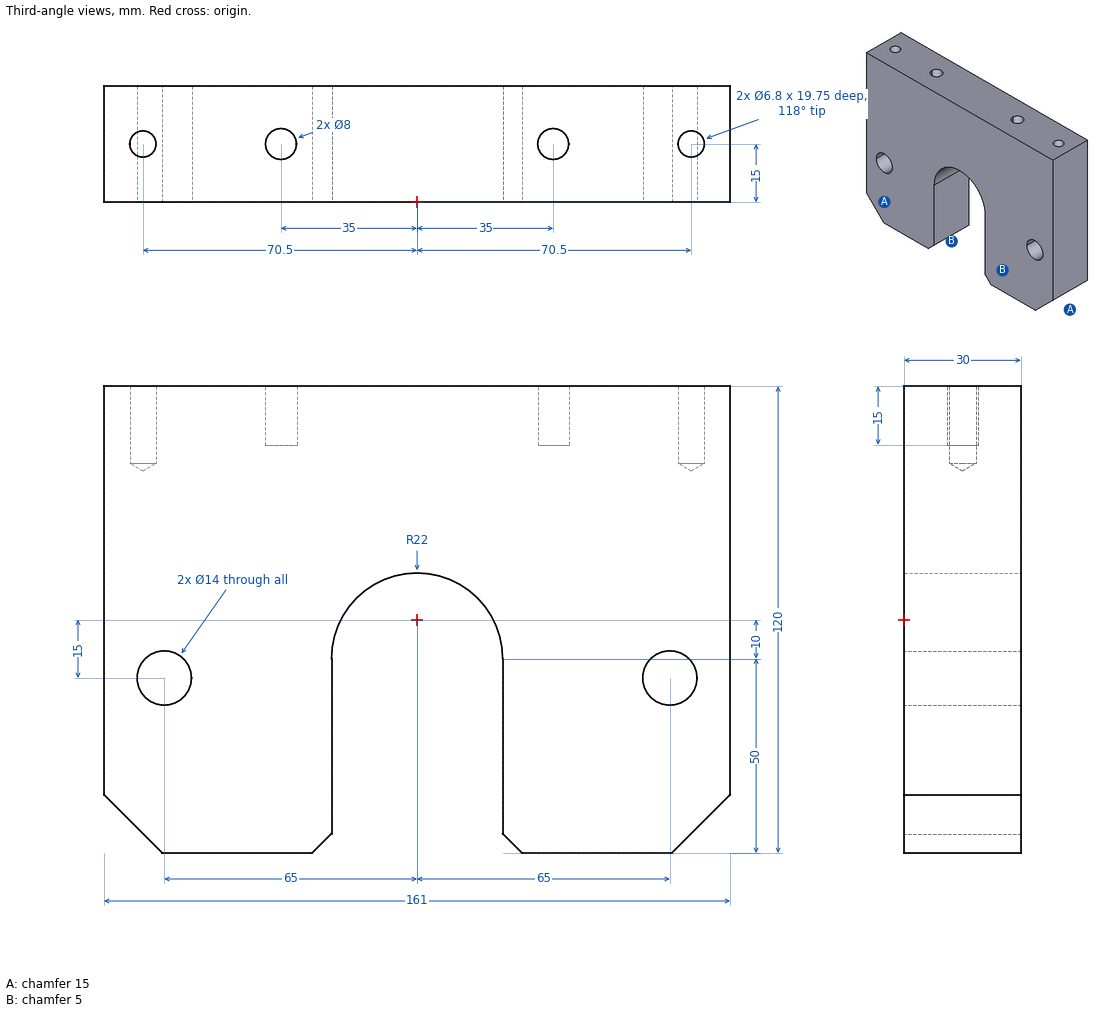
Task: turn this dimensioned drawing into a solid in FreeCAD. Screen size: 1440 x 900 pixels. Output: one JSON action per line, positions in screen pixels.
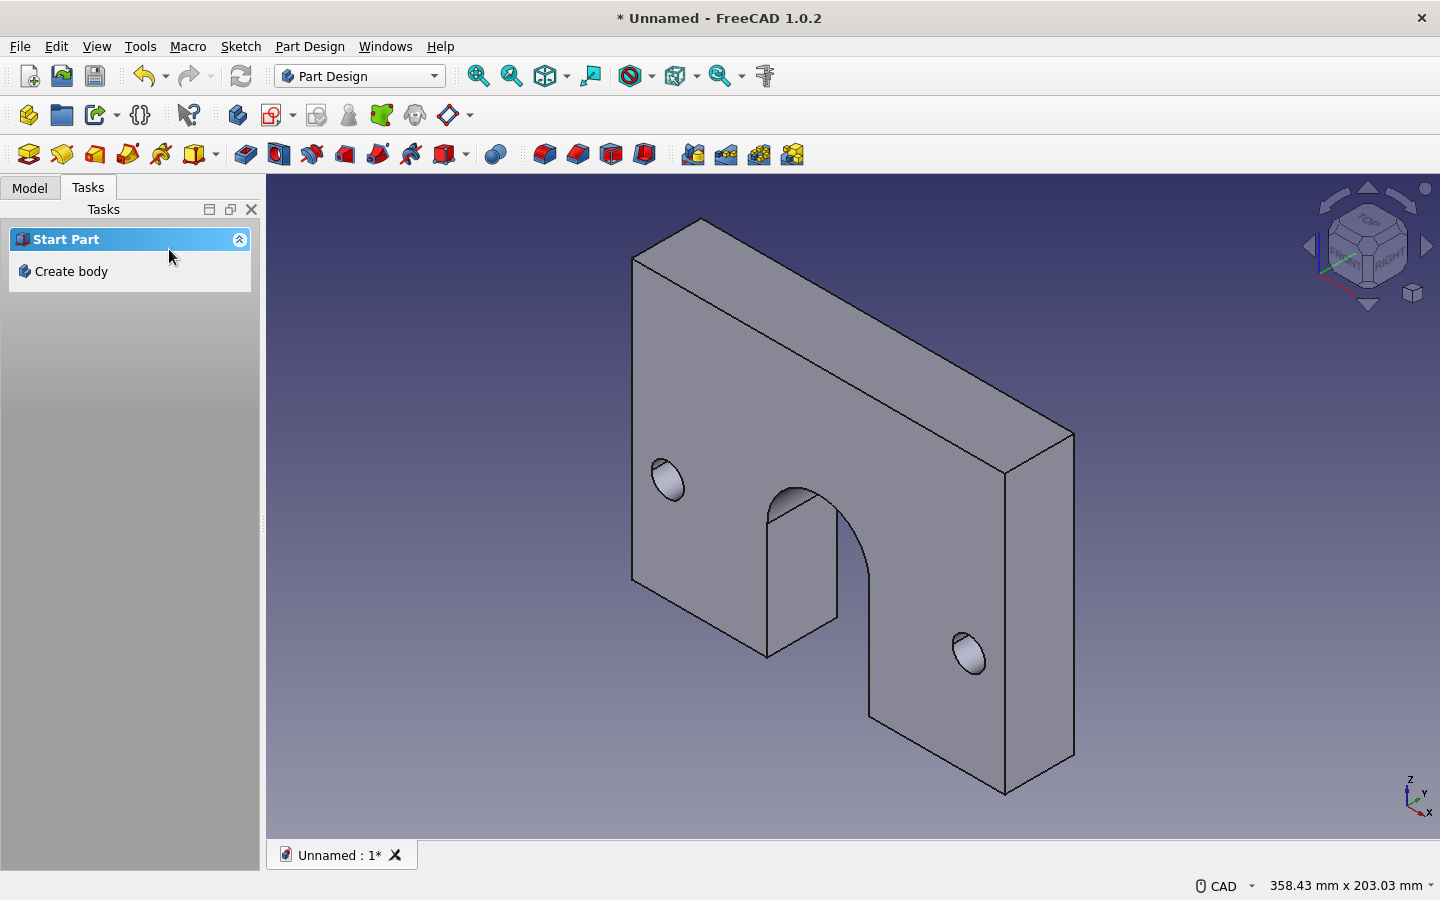
{"action": "left_click", "coordinate": [960, 407]}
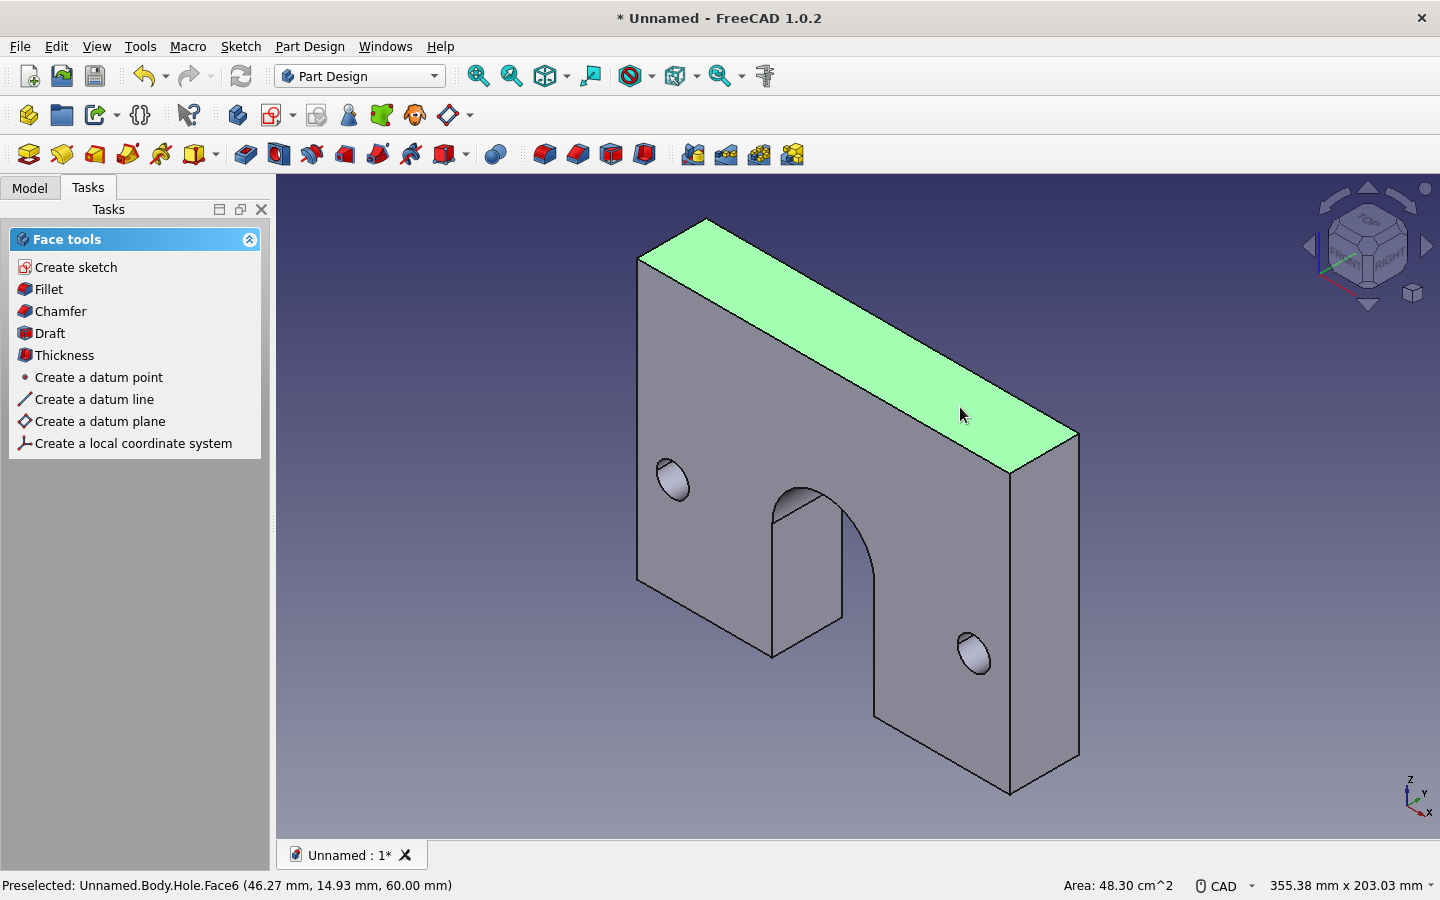
{"action": "left_click", "coordinate": [270, 116]}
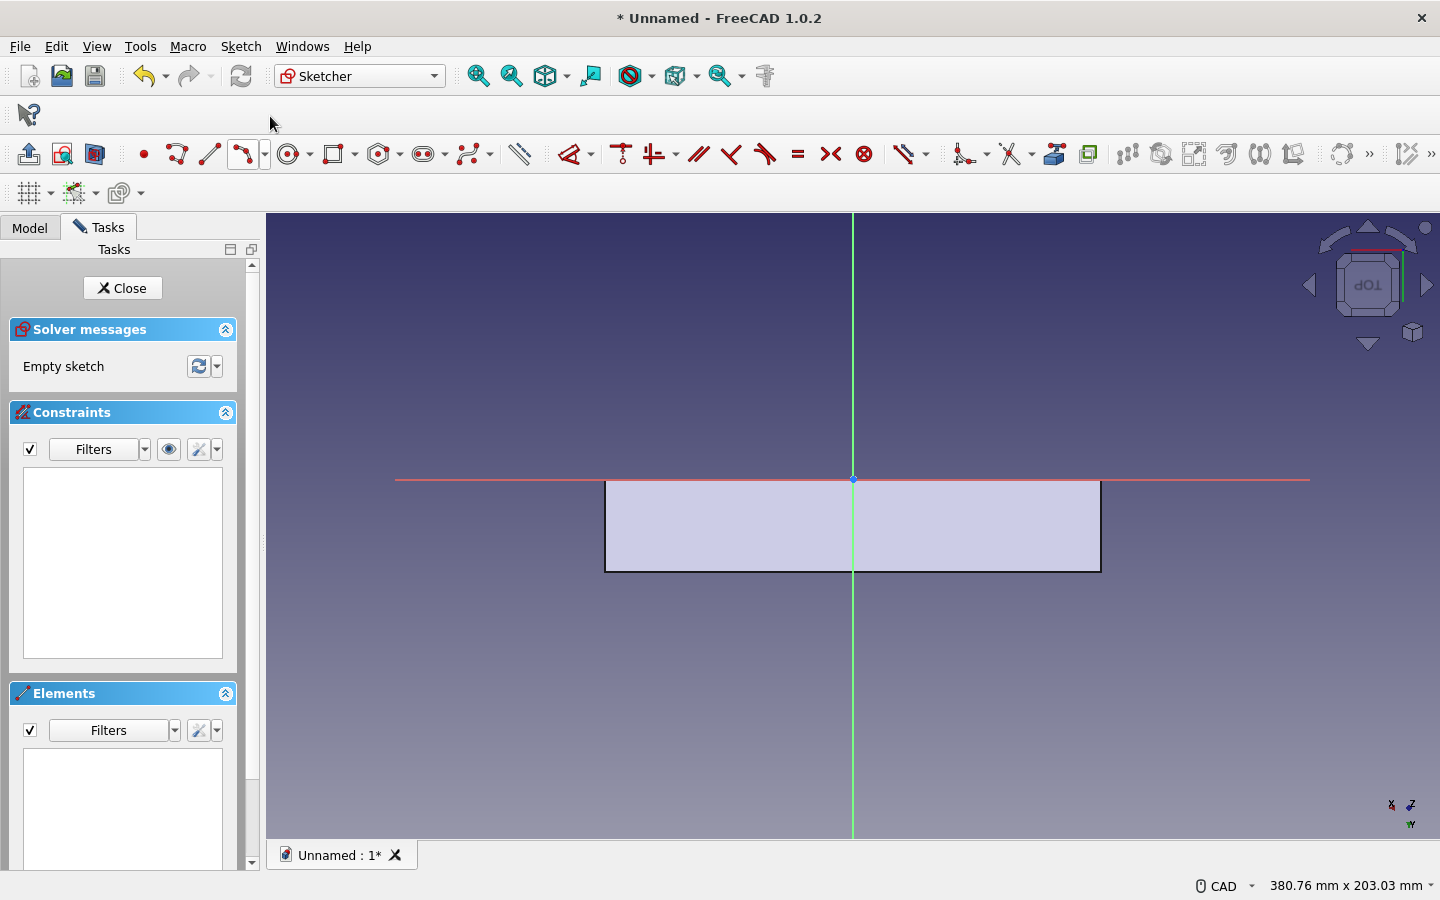
{"action": "scroll", "coordinate": [992, 472], "scroll_direction": "up", "scroll_amount": 2}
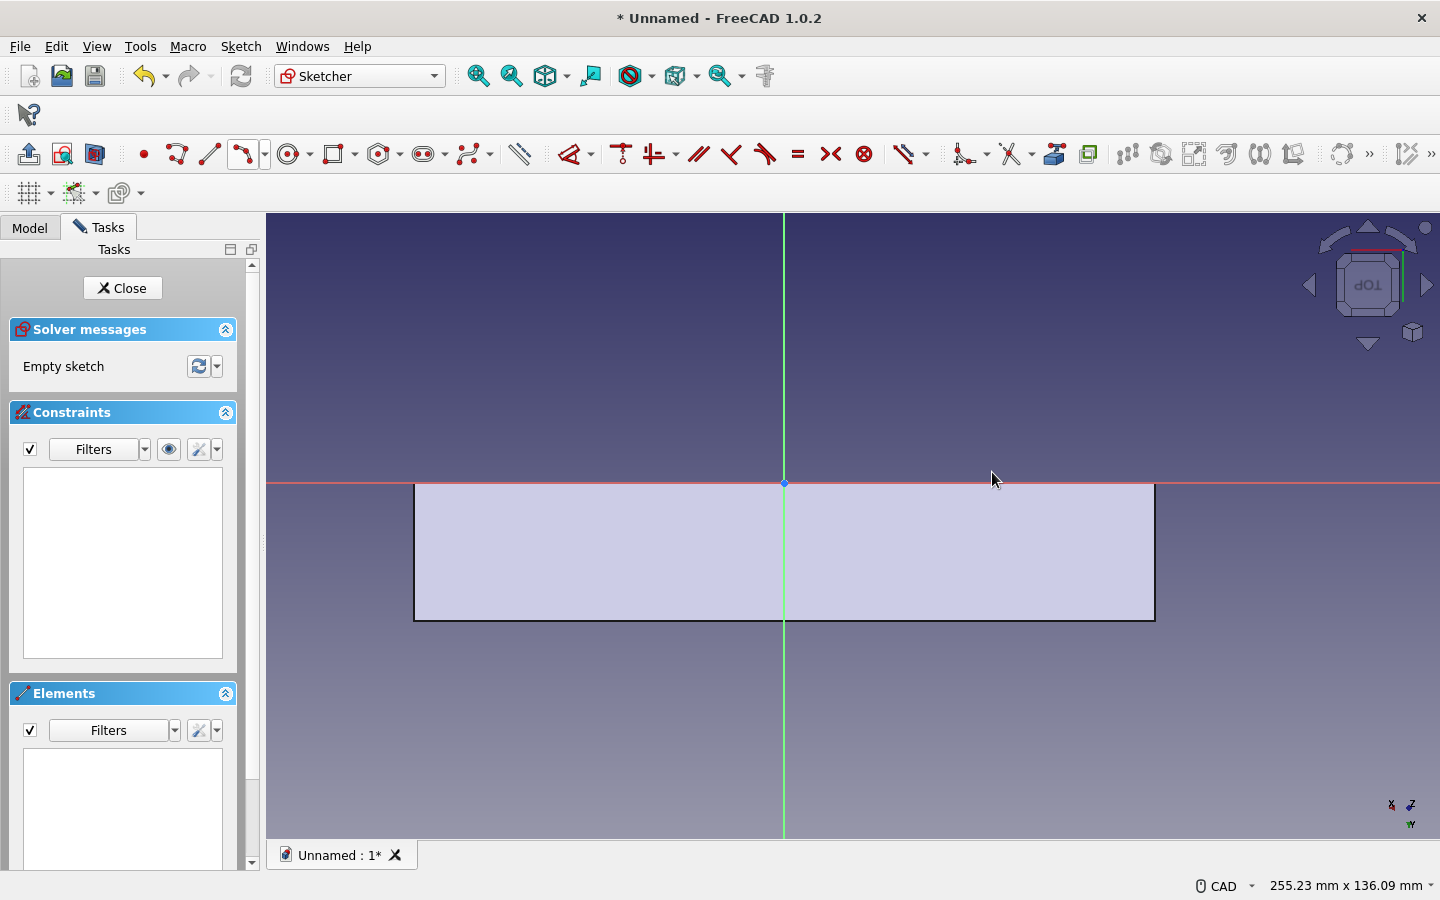
{"action": "key", "text": "g c"}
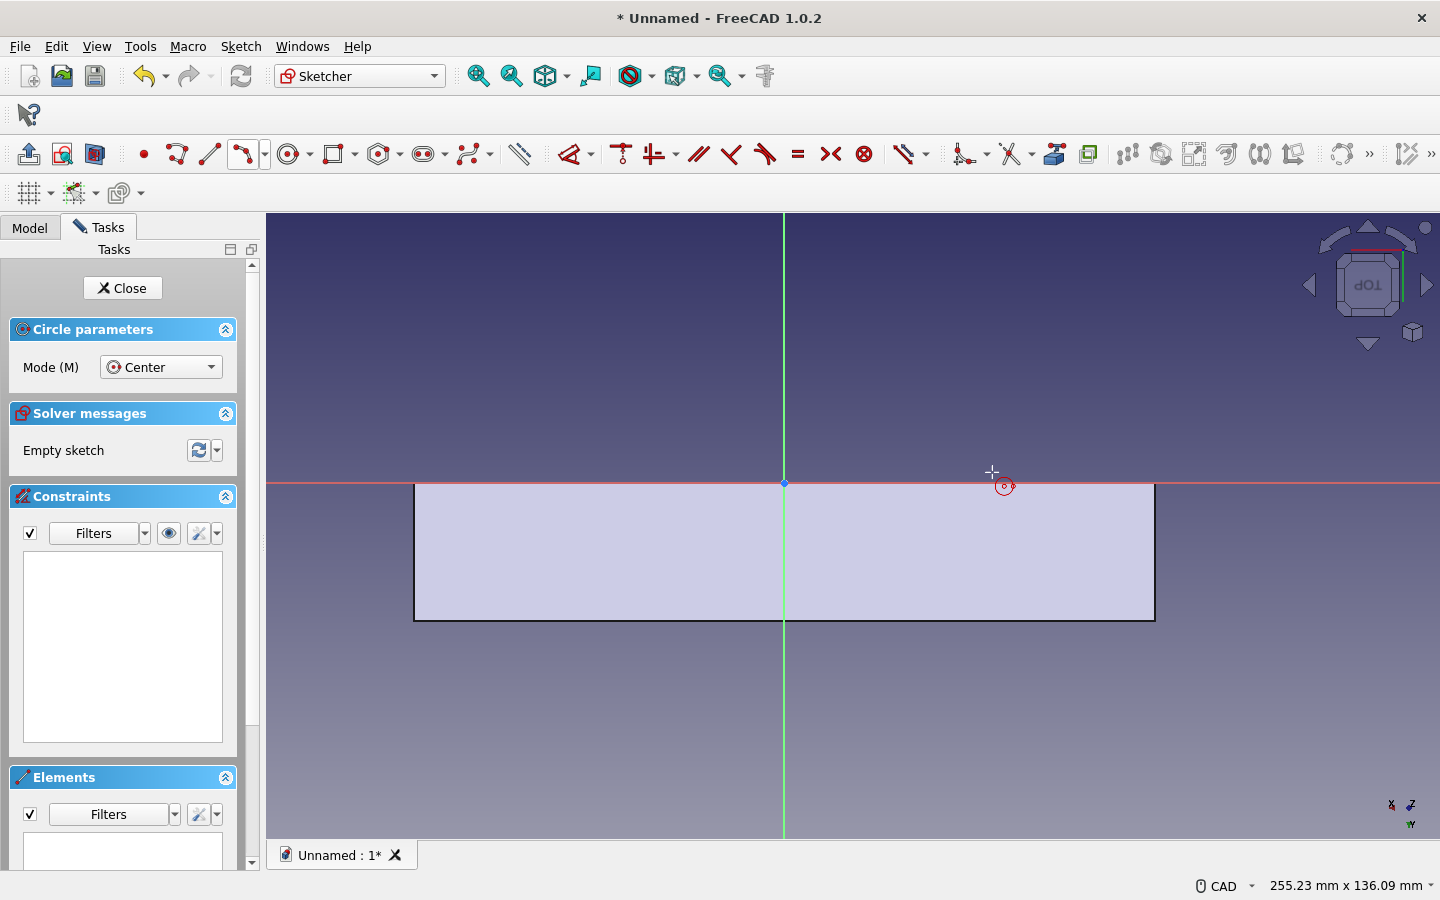
{"action": "scroll", "coordinate": [460, 552], "scroll_direction": "up", "scroll_amount": 2}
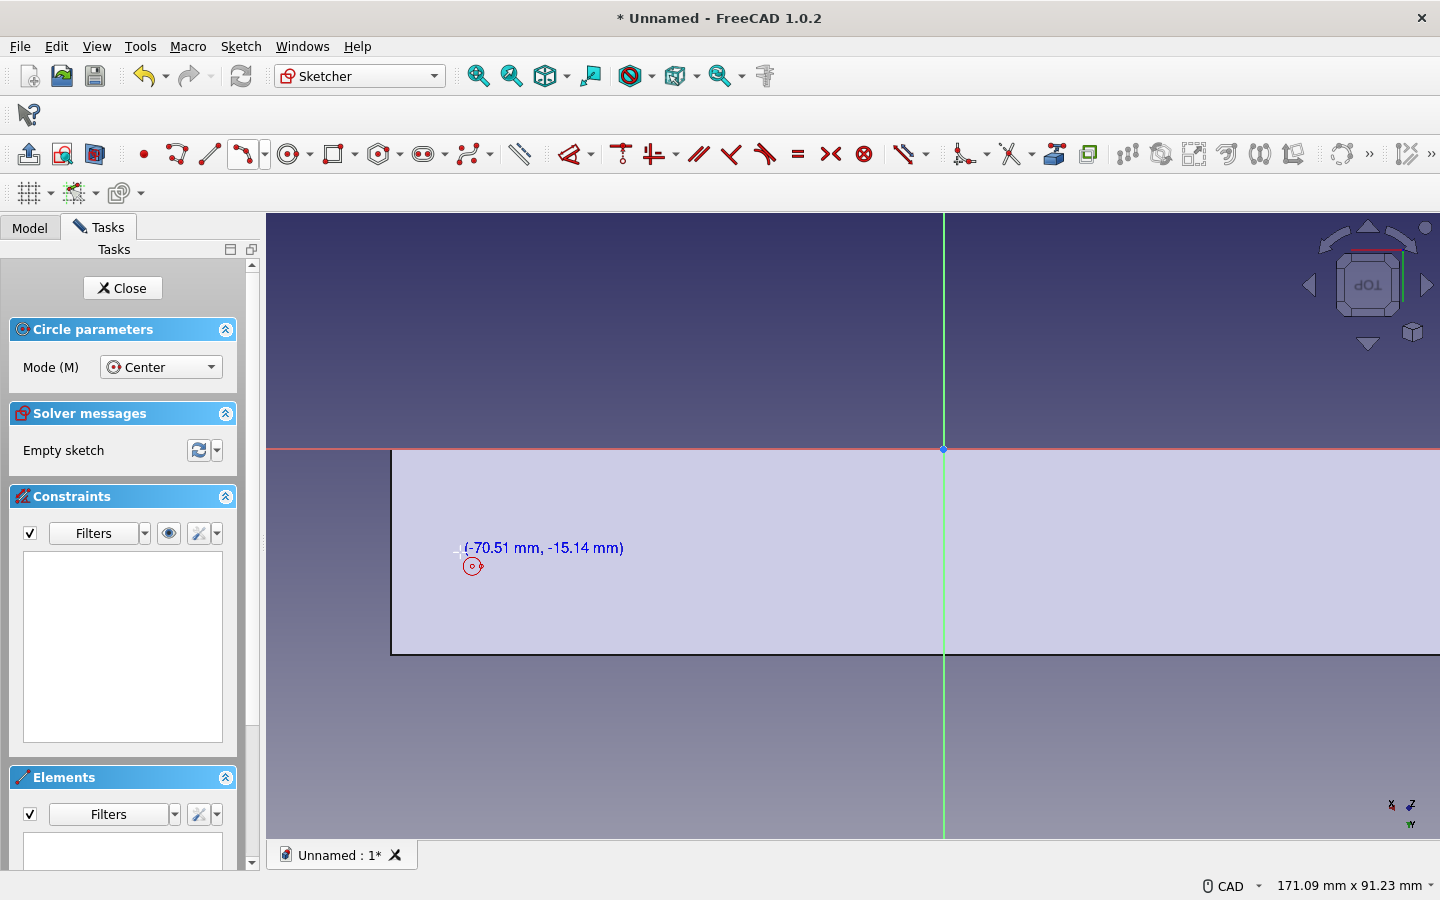
{"action": "left_click", "coordinate": [460, 552]}
{"action": "left_click", "coordinate": [476, 536]}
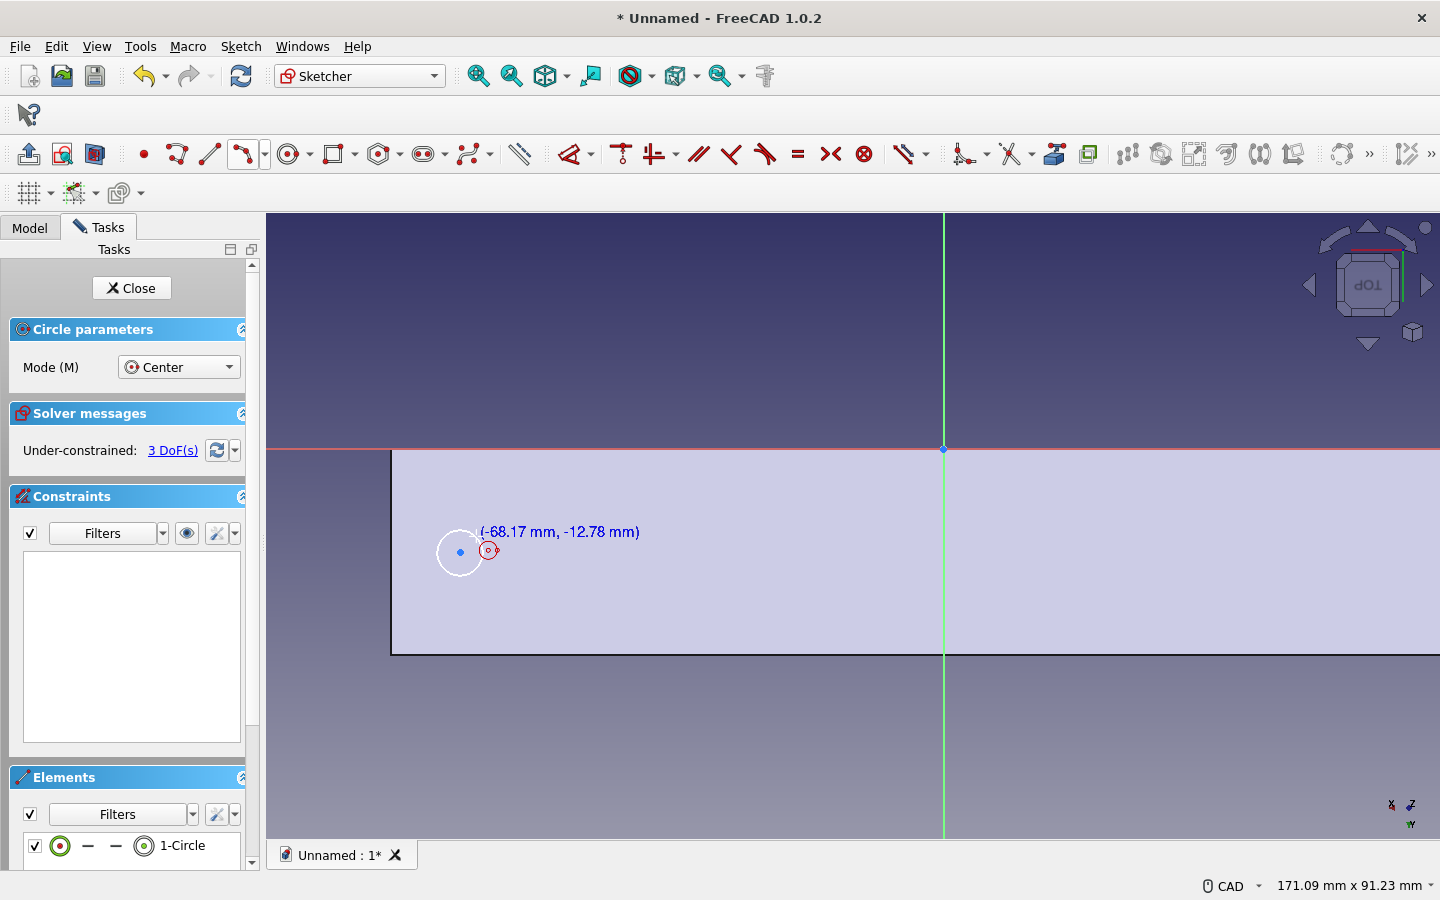
{"action": "scroll", "coordinate": [461, 554], "scroll_direction": "down", "scroll_amount": 2}